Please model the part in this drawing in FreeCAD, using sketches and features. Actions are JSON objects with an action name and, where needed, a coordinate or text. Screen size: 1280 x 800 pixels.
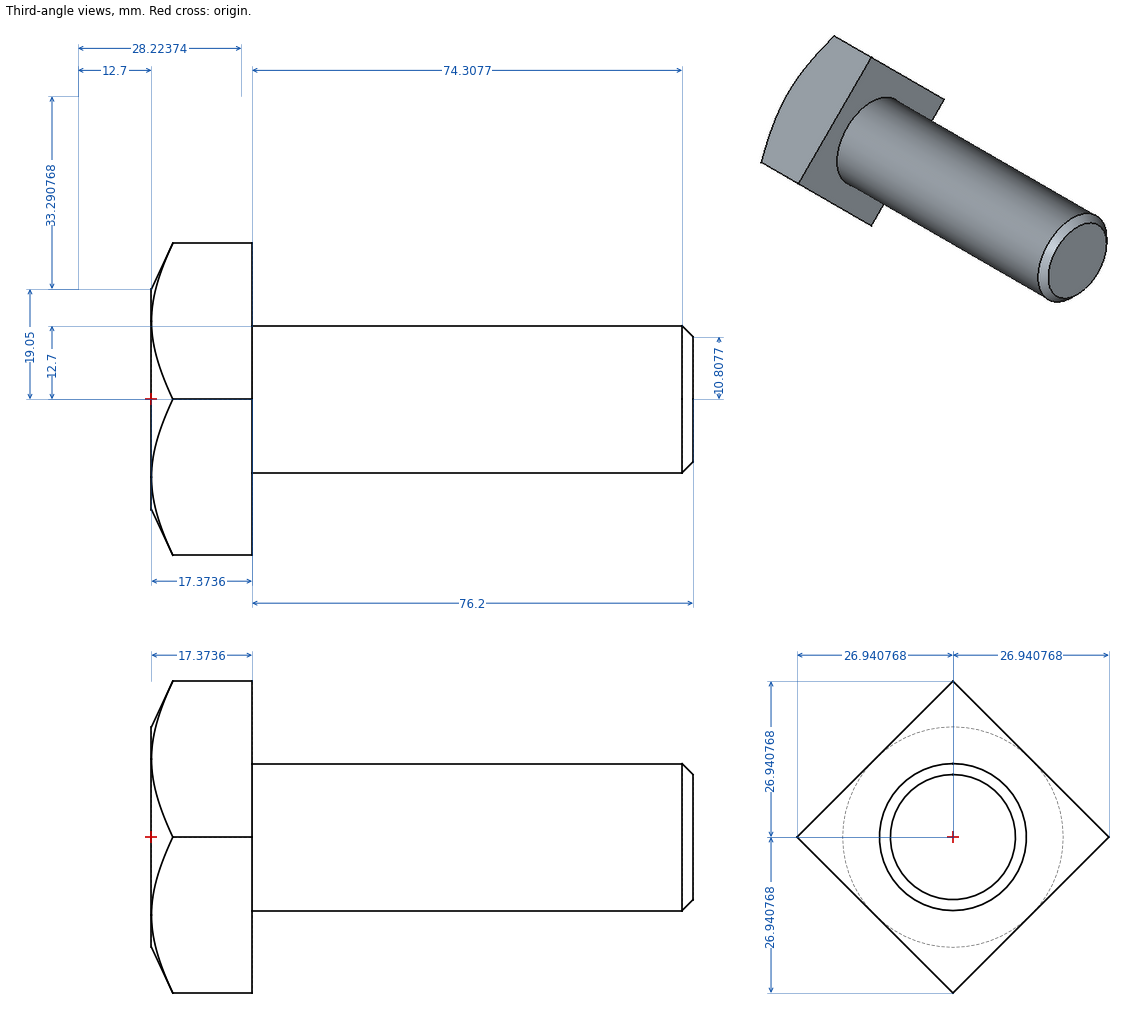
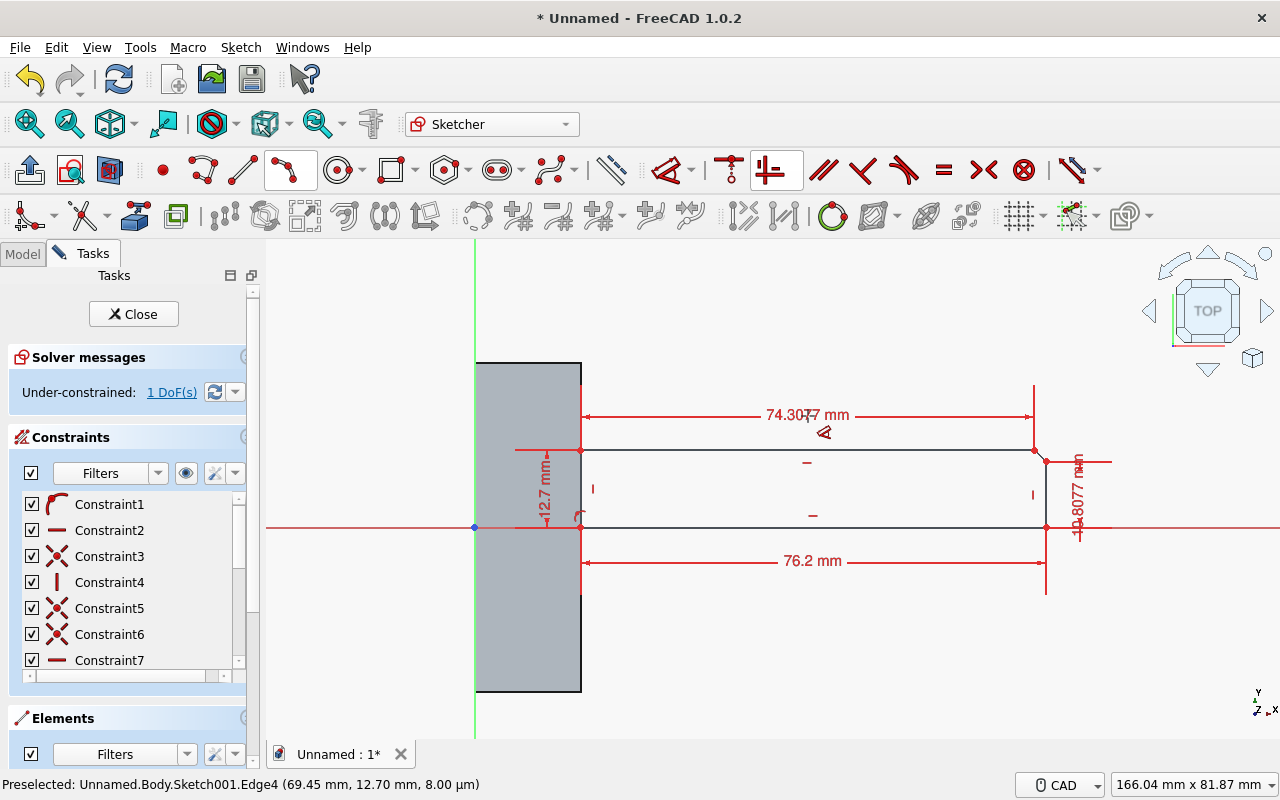
{"action": "left_click", "coordinate": [581, 528]}
{"action": "left_click", "coordinate": [528, 562]}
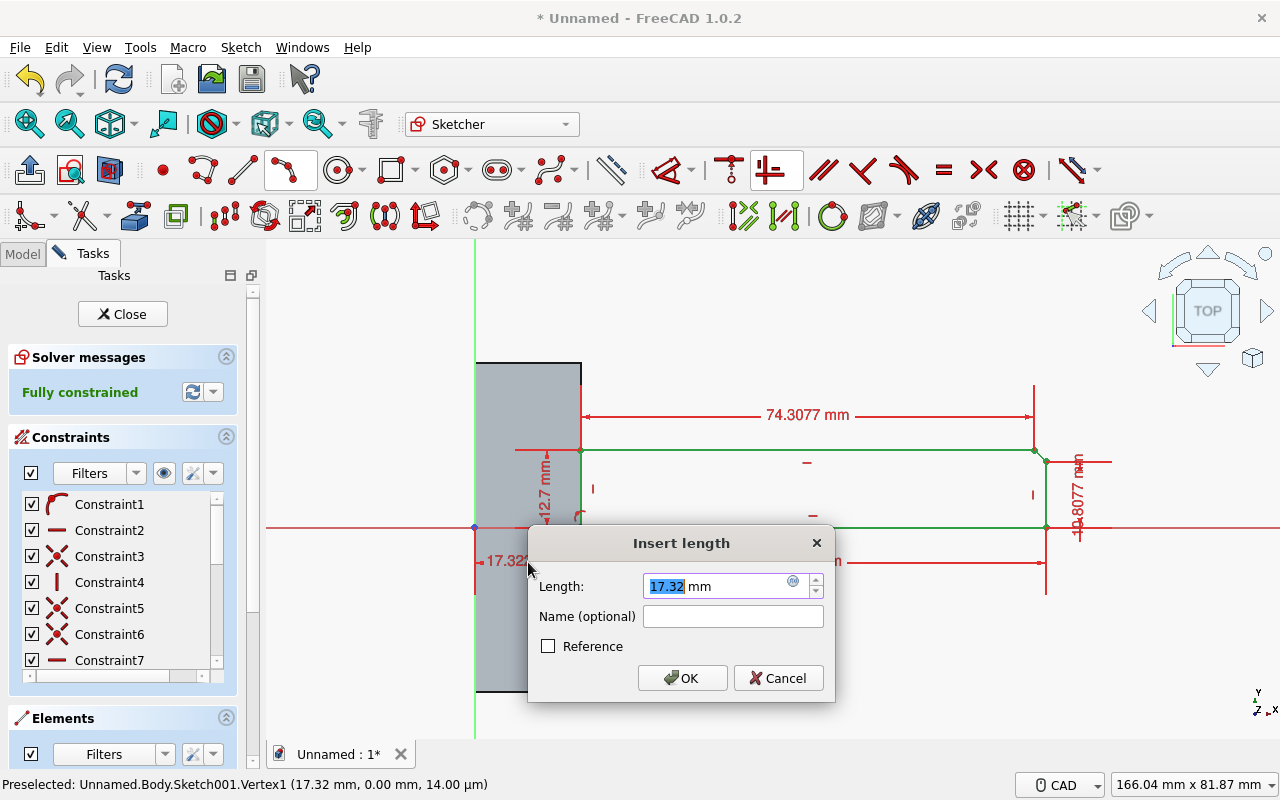
{"action": "type", "text": "17.3736"}
{"action": "key", "text": "Return"}
{"action": "key", "text": "Escape"}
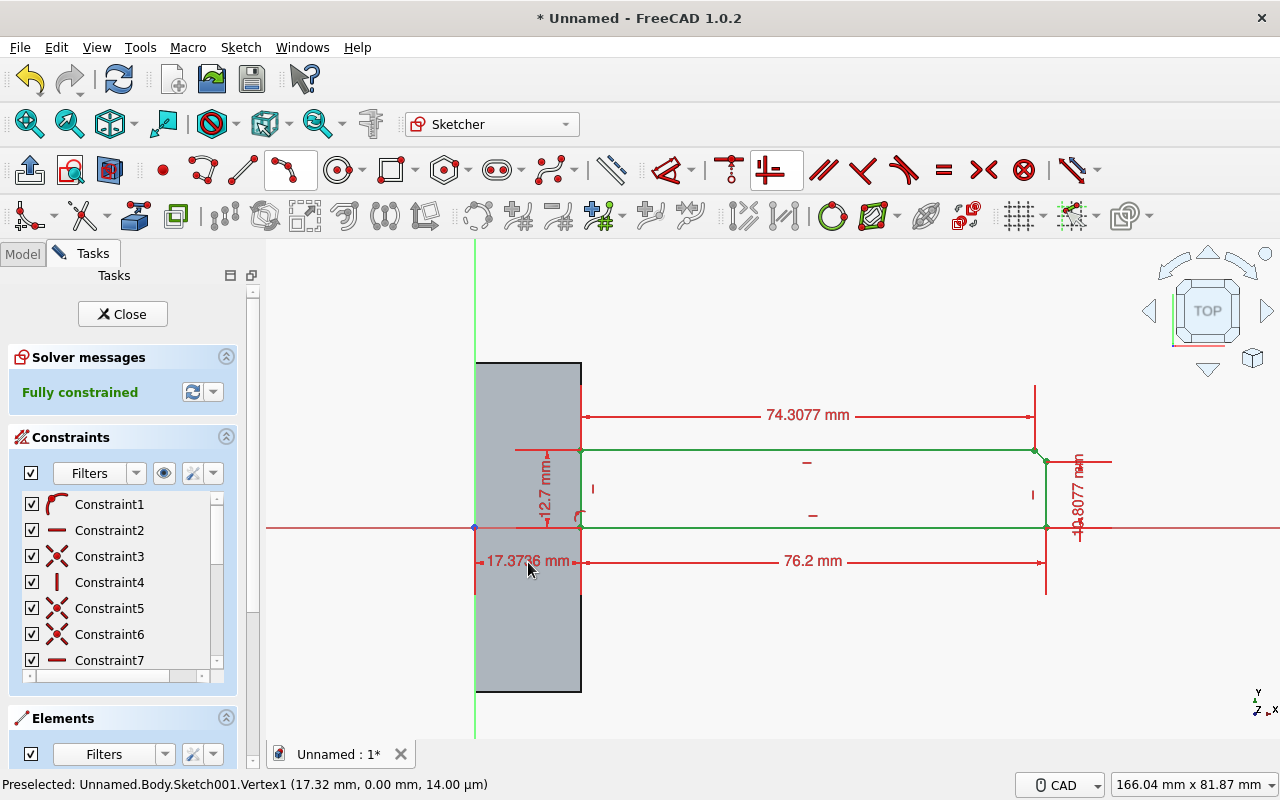
{"action": "left_click", "coordinate": [123, 314]}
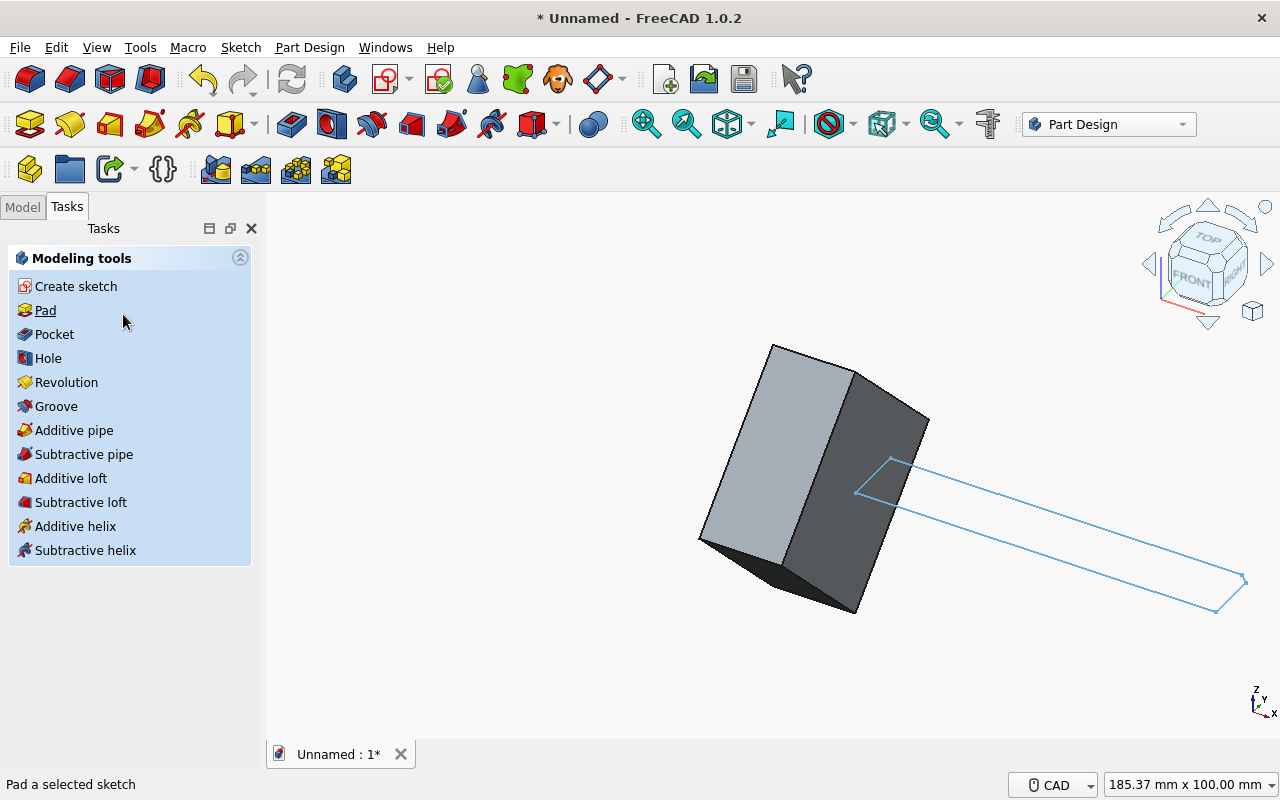
{"action": "left_click", "coordinate": [70, 124]}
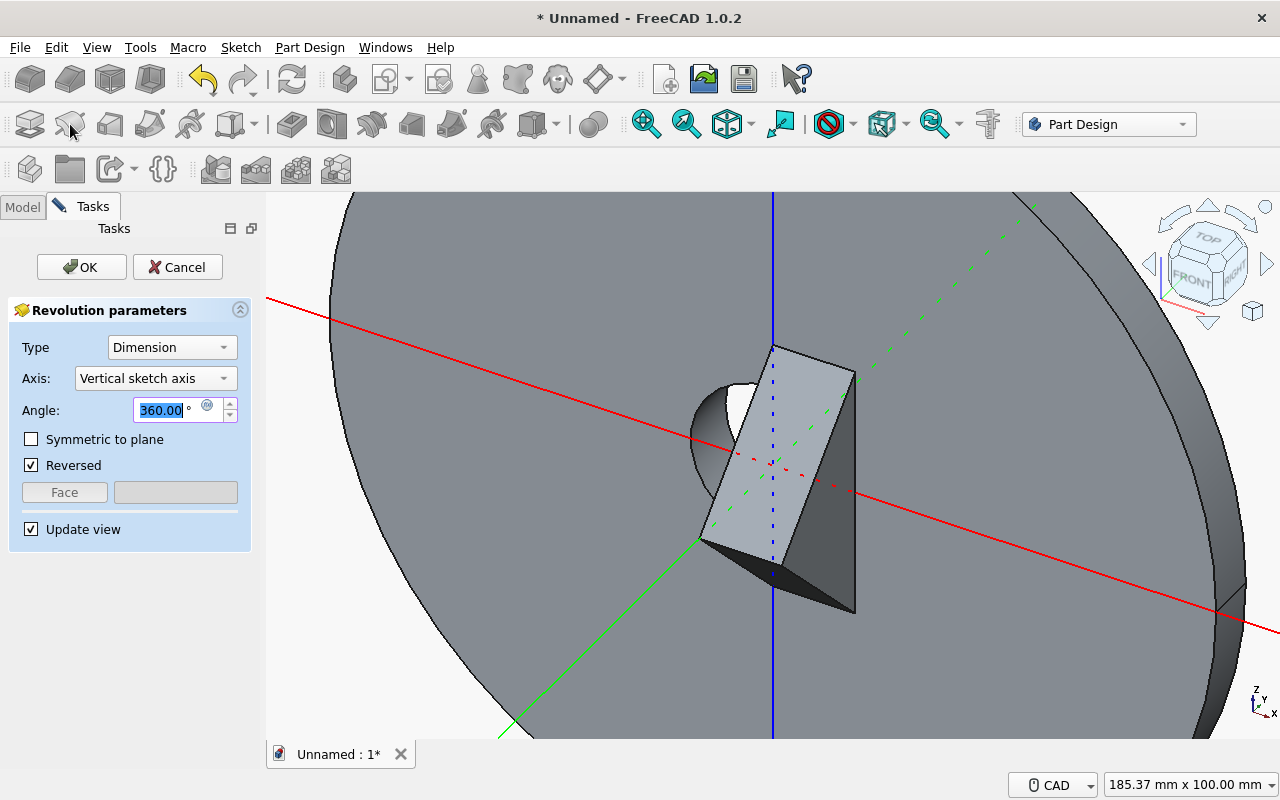
{"action": "left_click", "coordinate": [156, 378]}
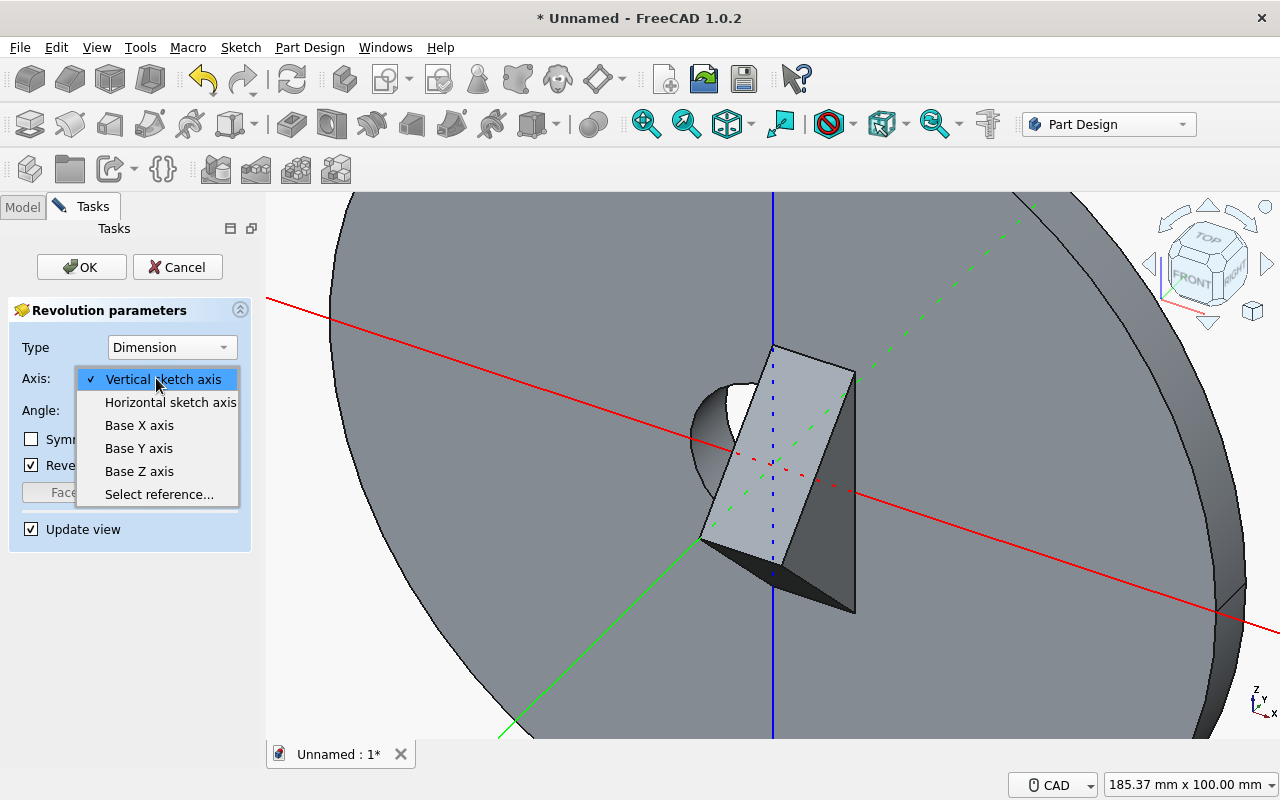
{"action": "left_click", "coordinate": [156, 402]}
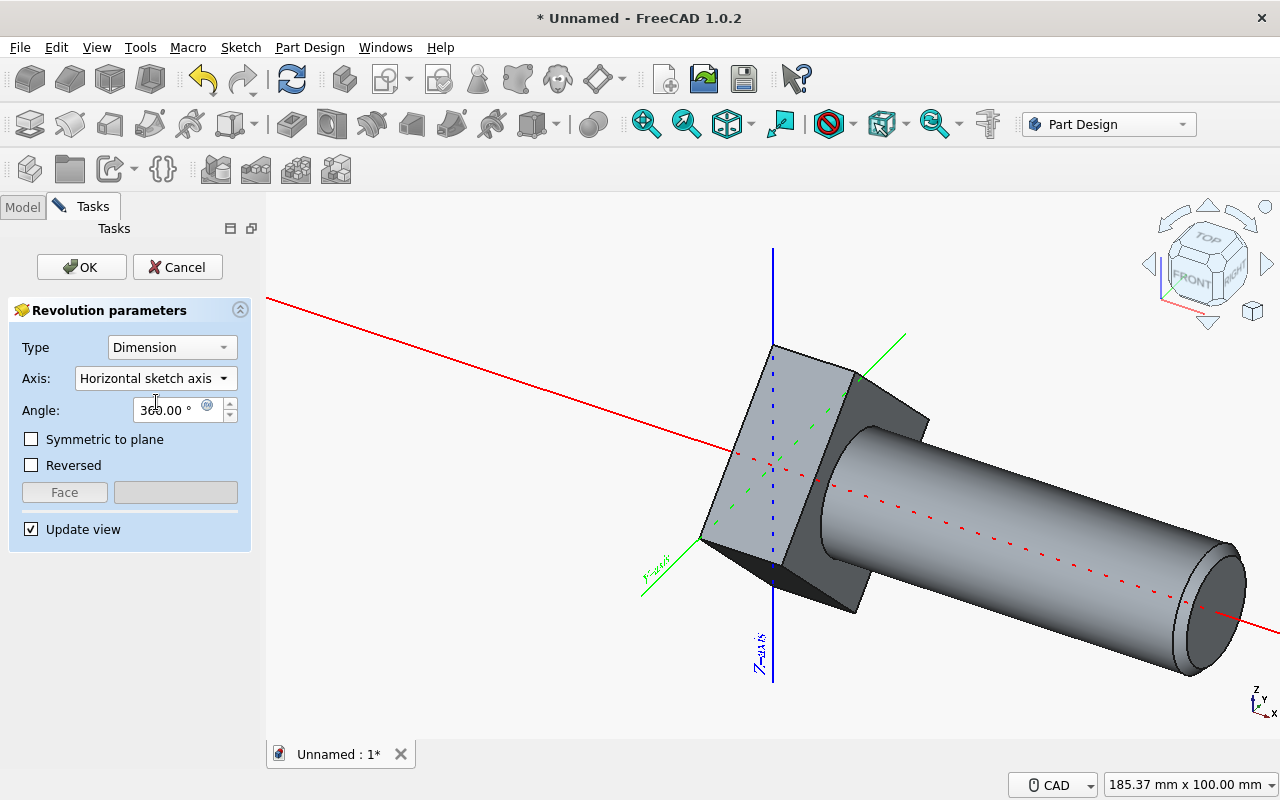
{"action": "left_click", "coordinate": [82, 267]}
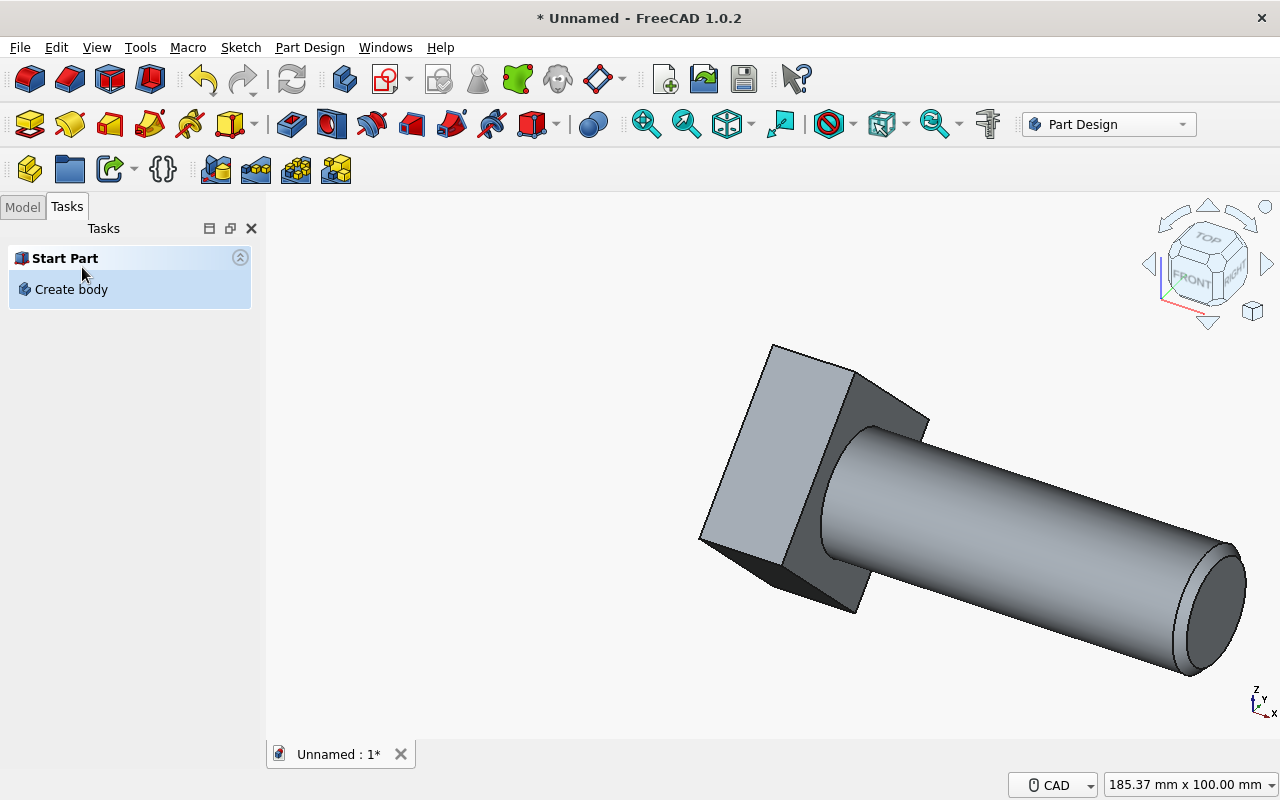
{"action": "key", "text": "v f"}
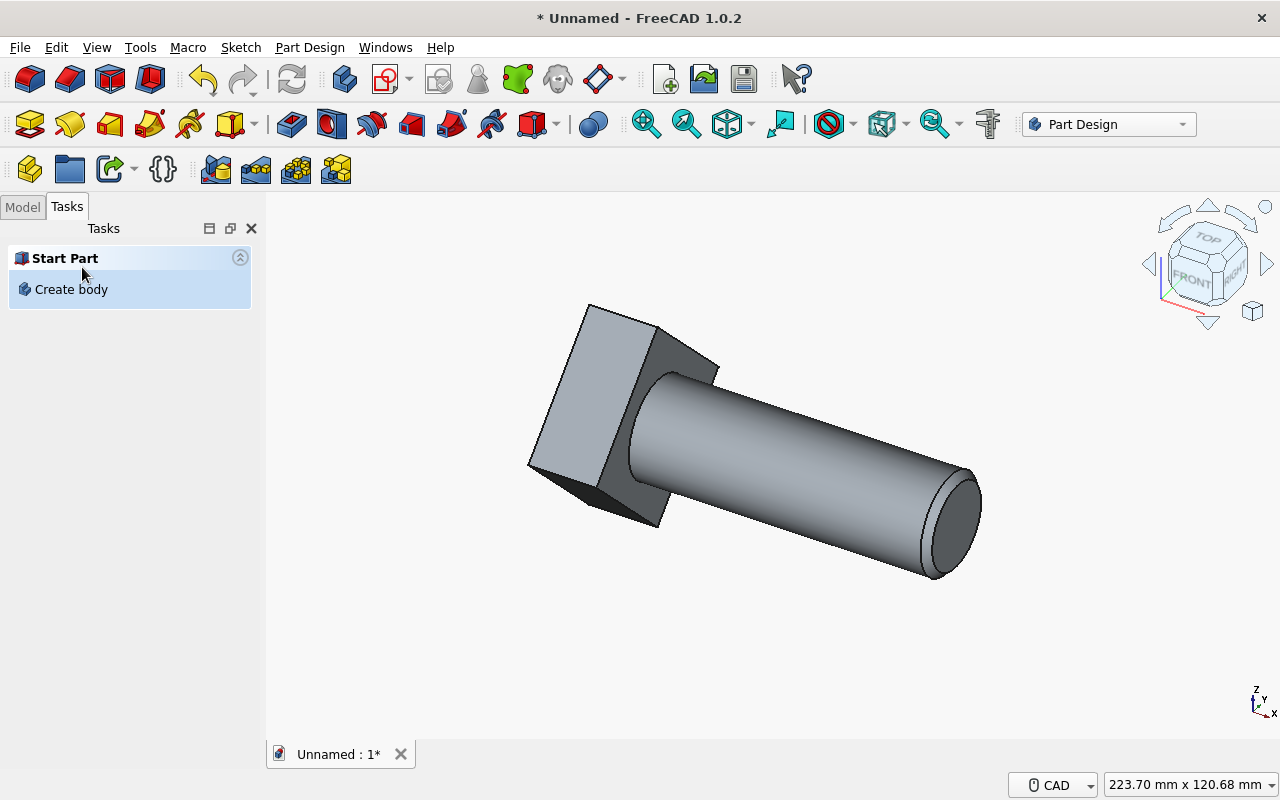
{"action": "left_click", "coordinate": [386, 80]}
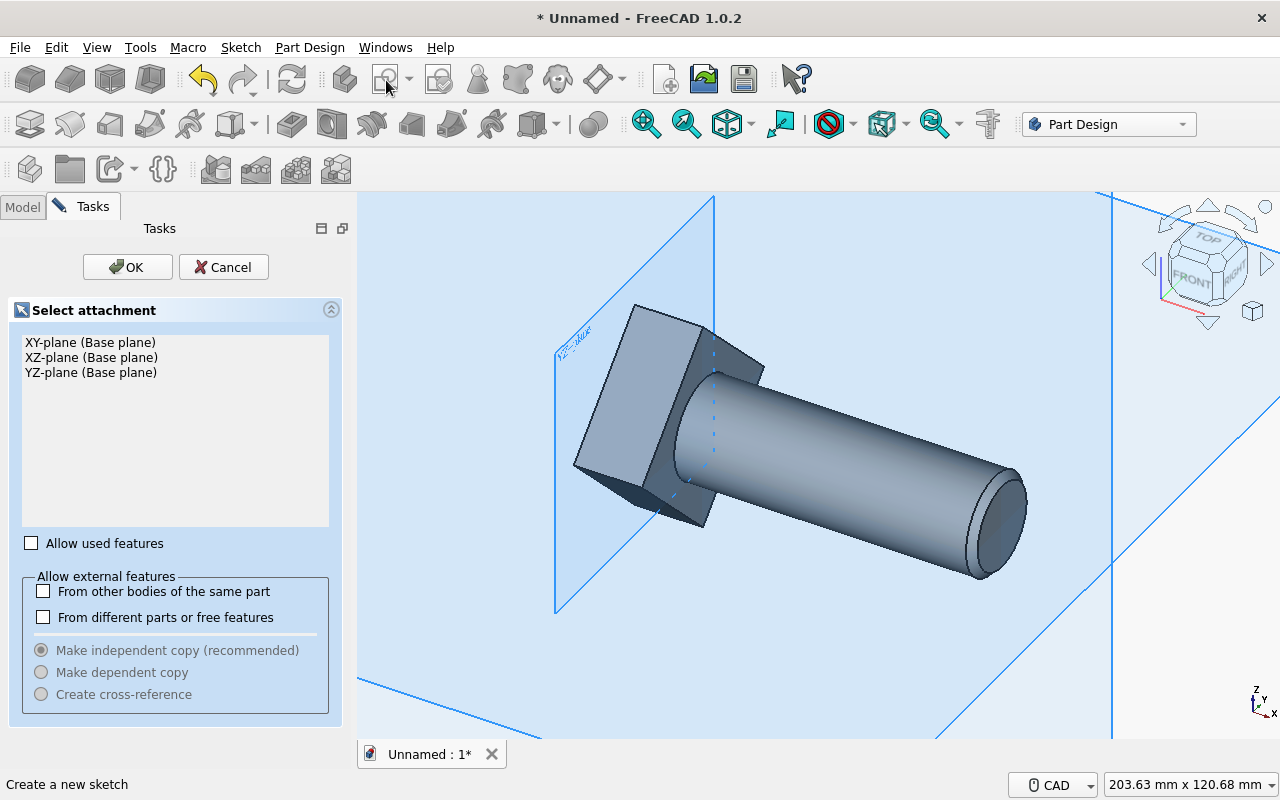
{"action": "left_click", "coordinate": [82, 342]}